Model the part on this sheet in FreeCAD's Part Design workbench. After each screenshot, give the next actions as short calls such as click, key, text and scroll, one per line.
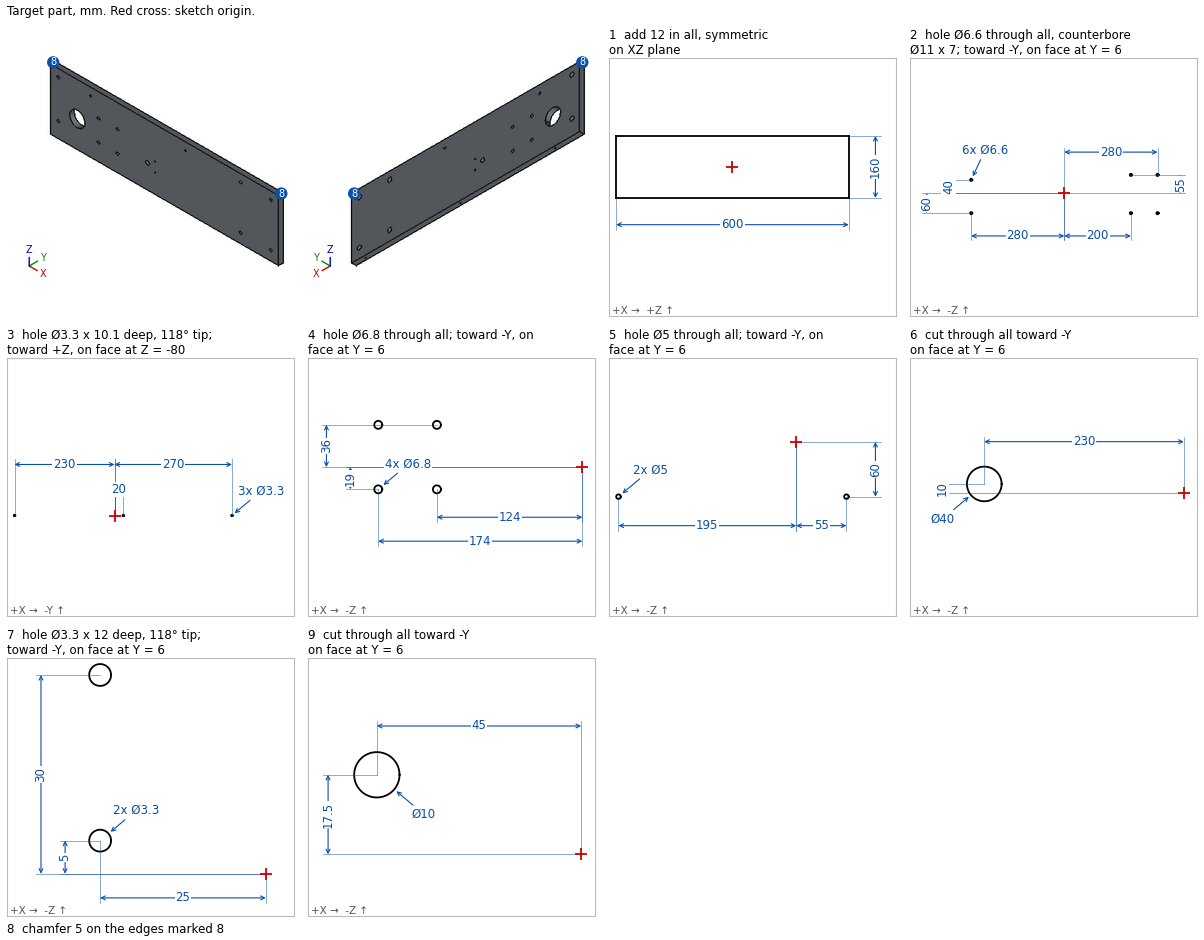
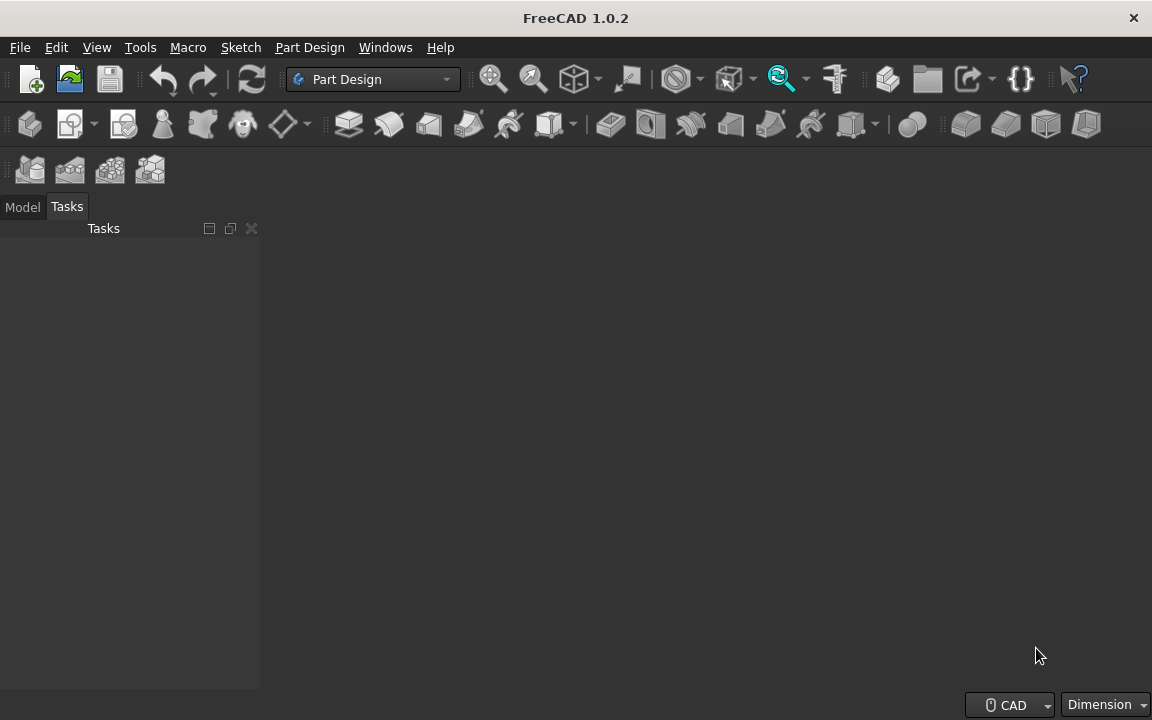
key(ctrl+n)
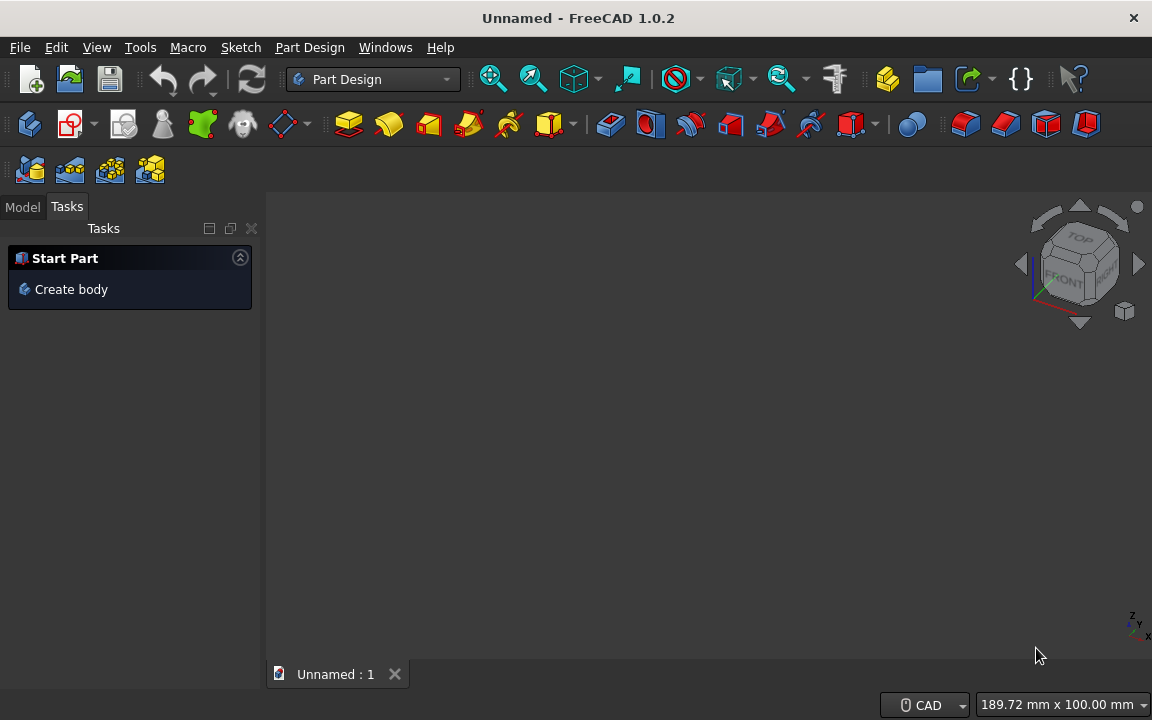
click(70, 124)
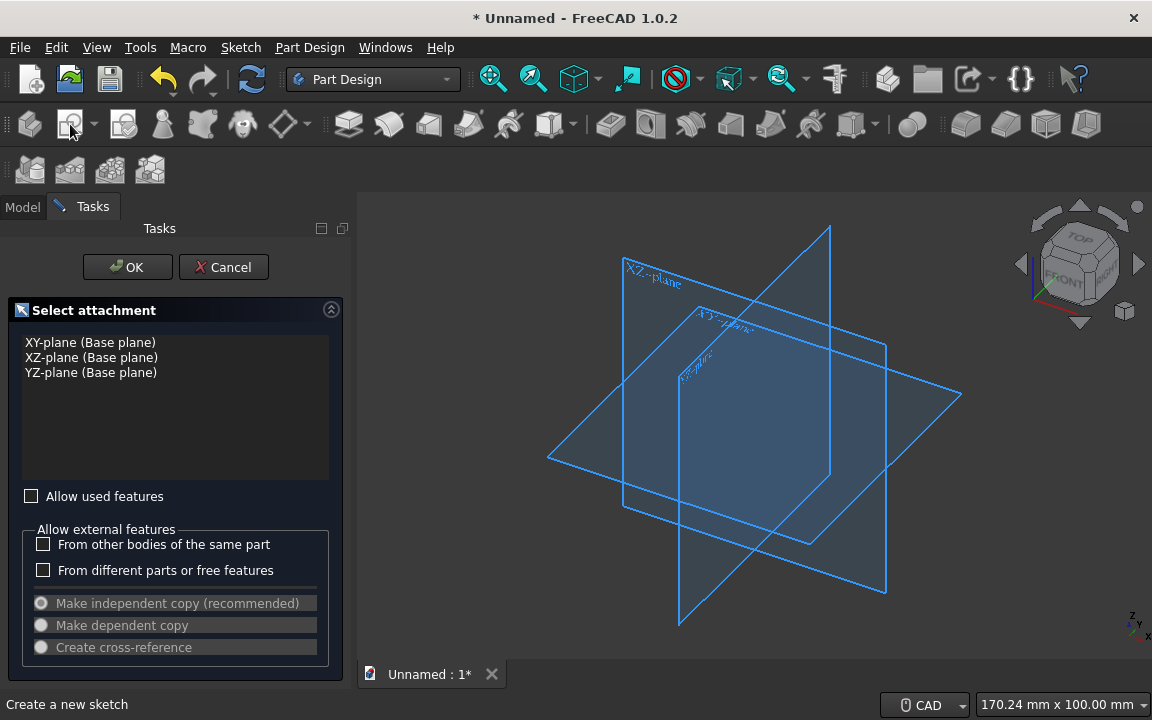
click(82, 358)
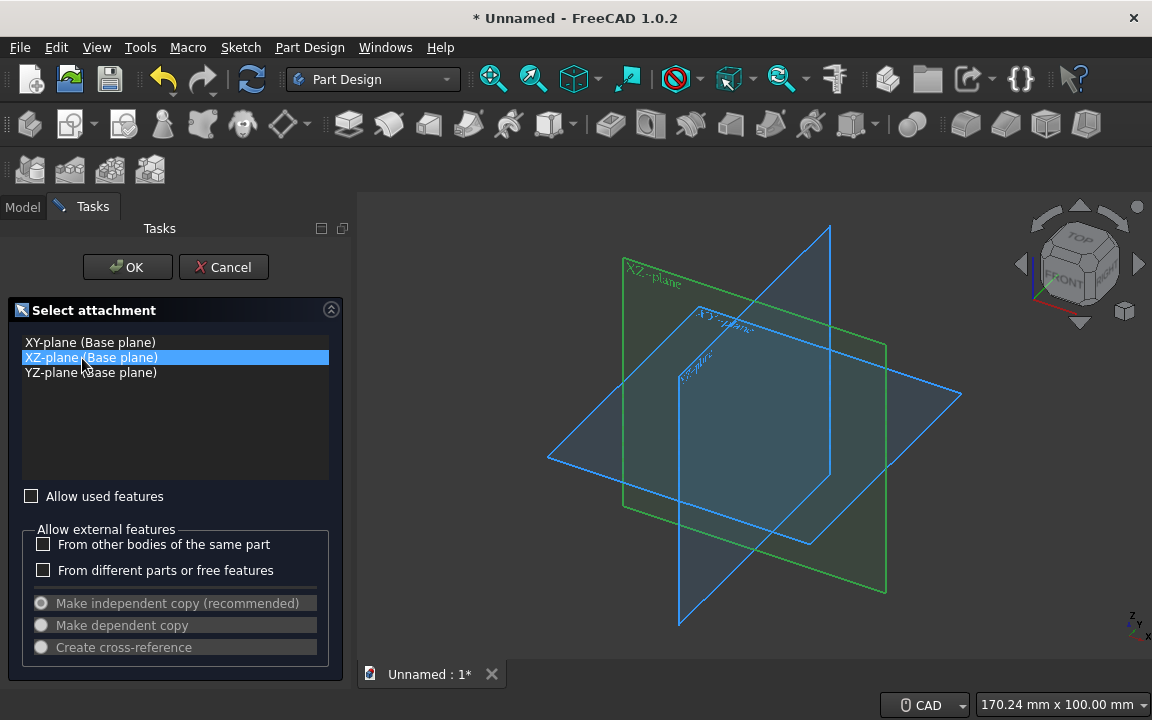
click(128, 267)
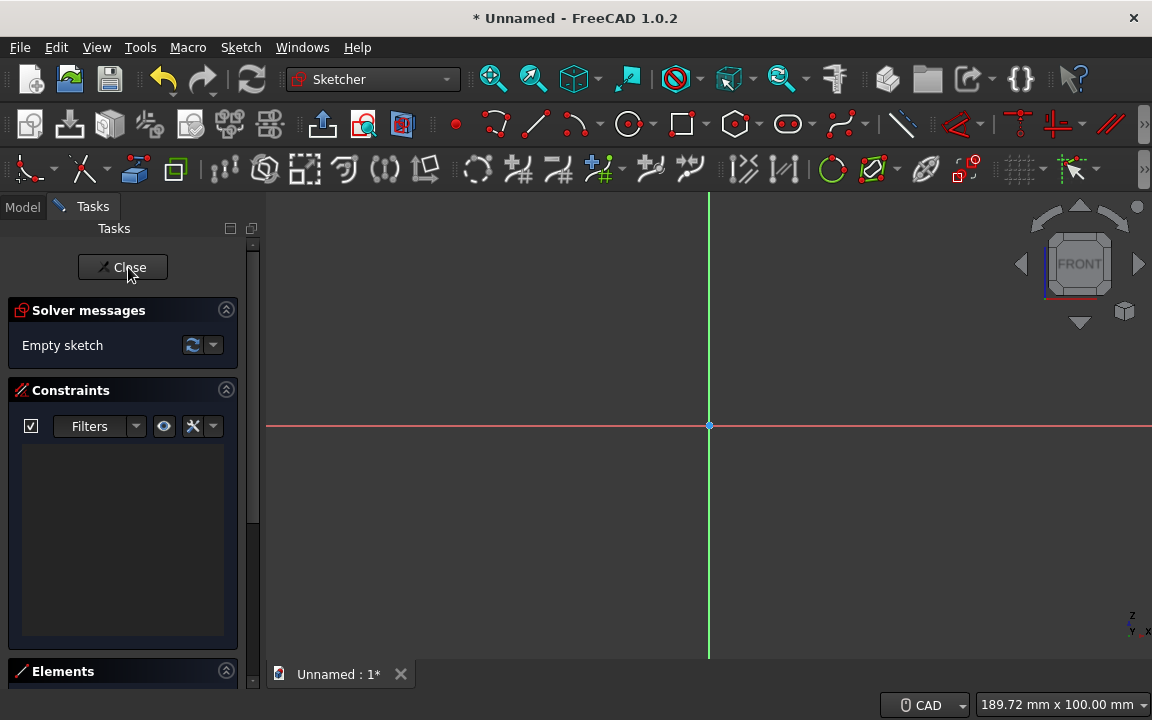
scroll(627, 426, down, 9)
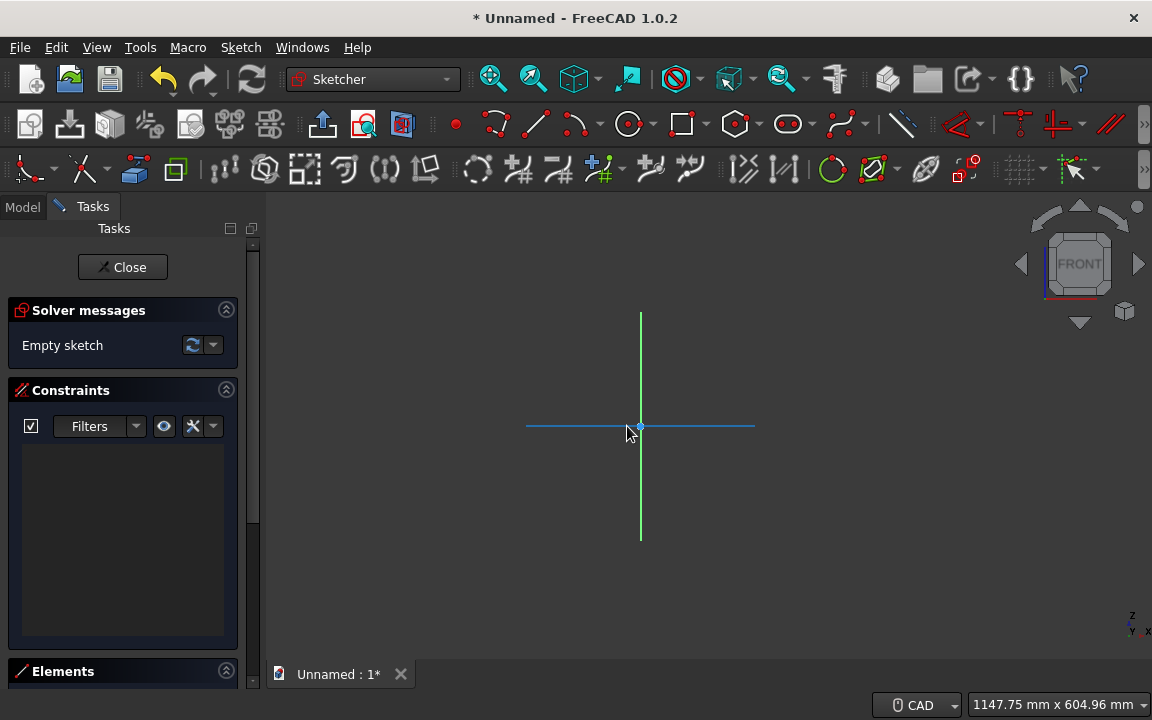
key(g)
key(v)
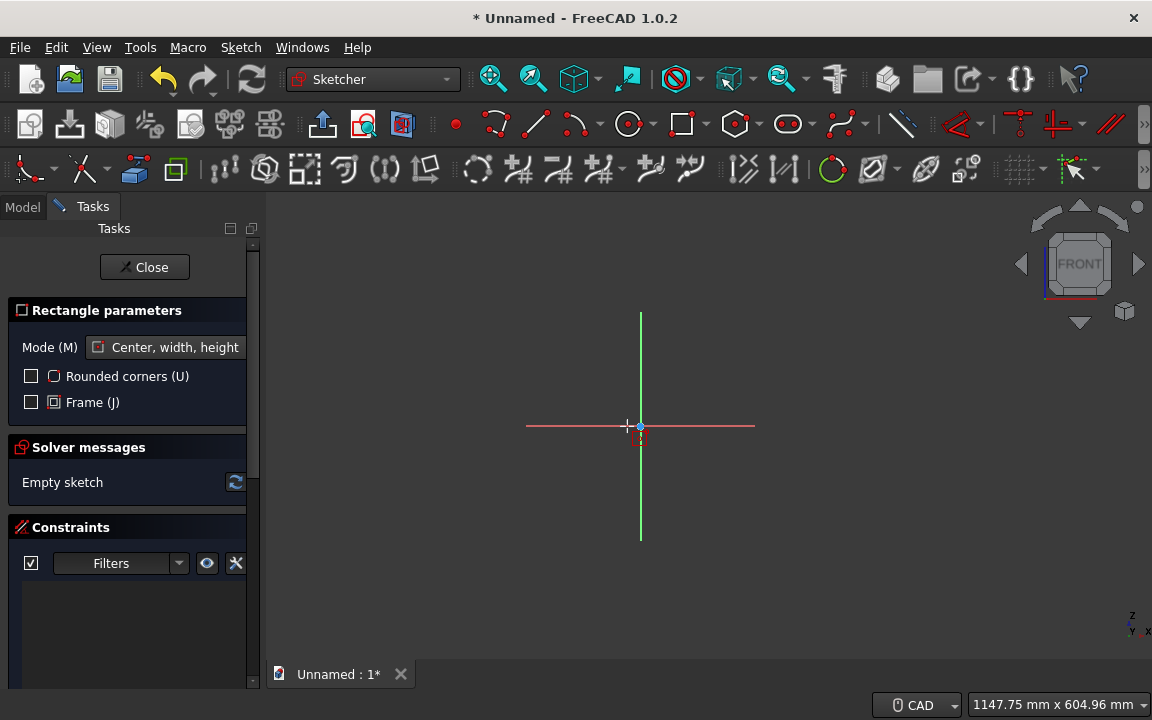
click(641, 426)
move(872, 365)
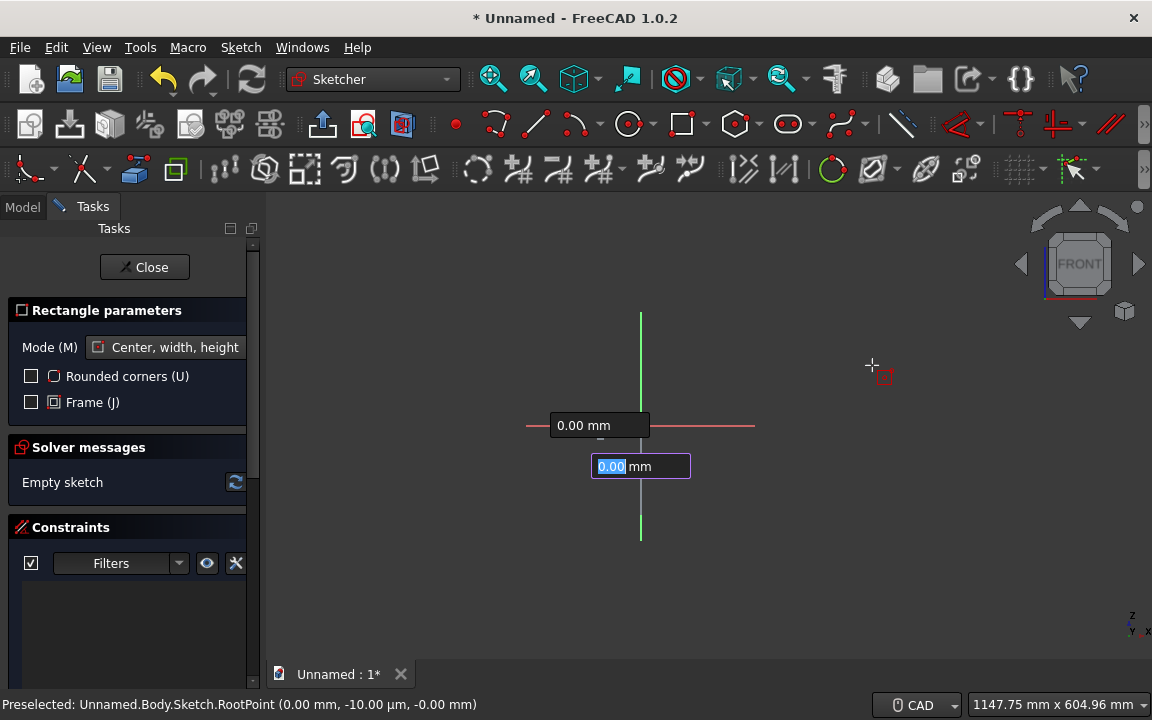
text(600)
key(Tab)
text(160)
key(Return)
key(Escape)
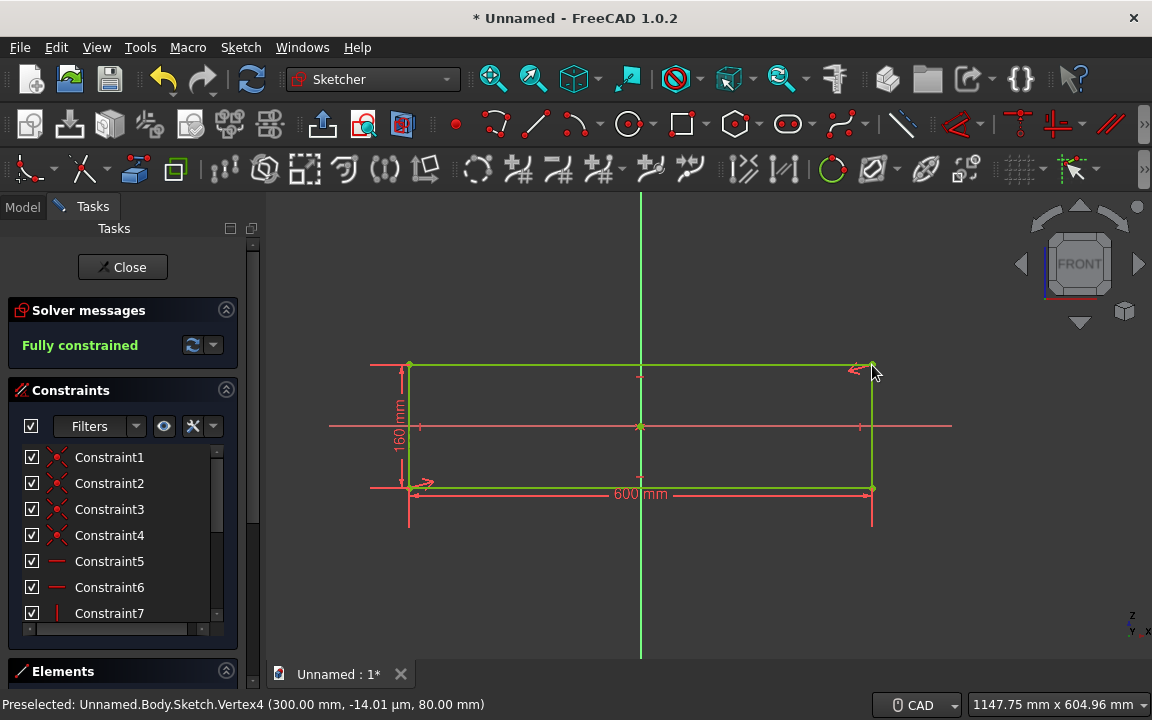
click(123, 267)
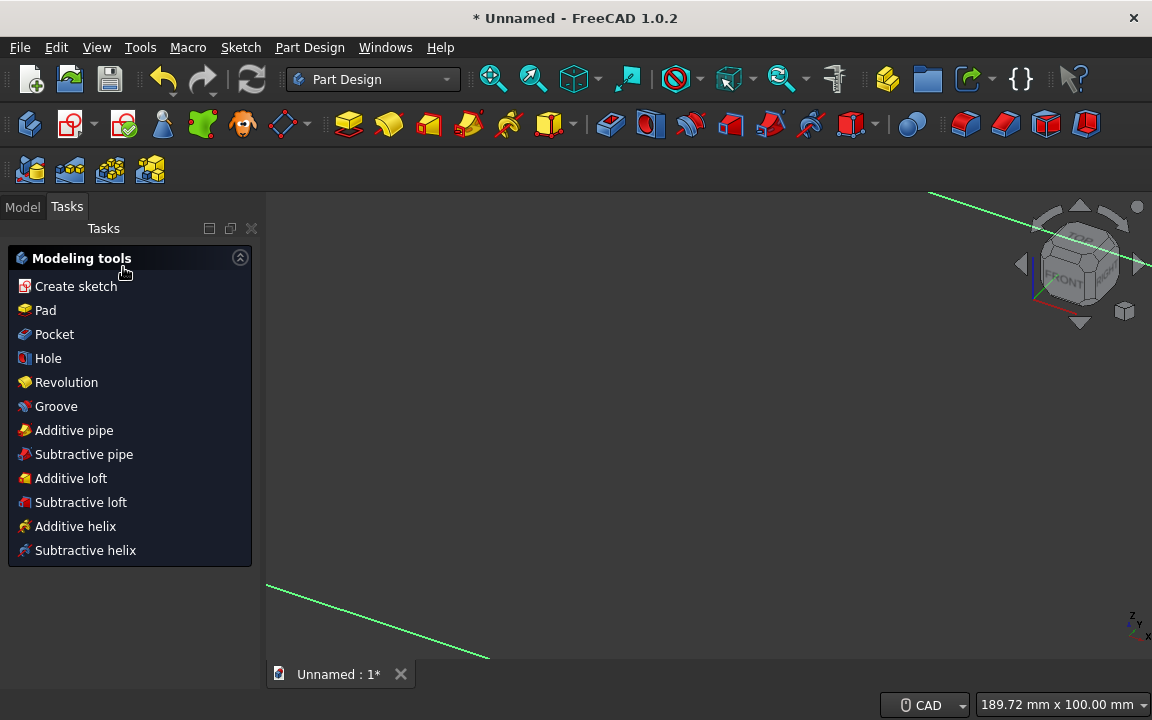
click(350, 124)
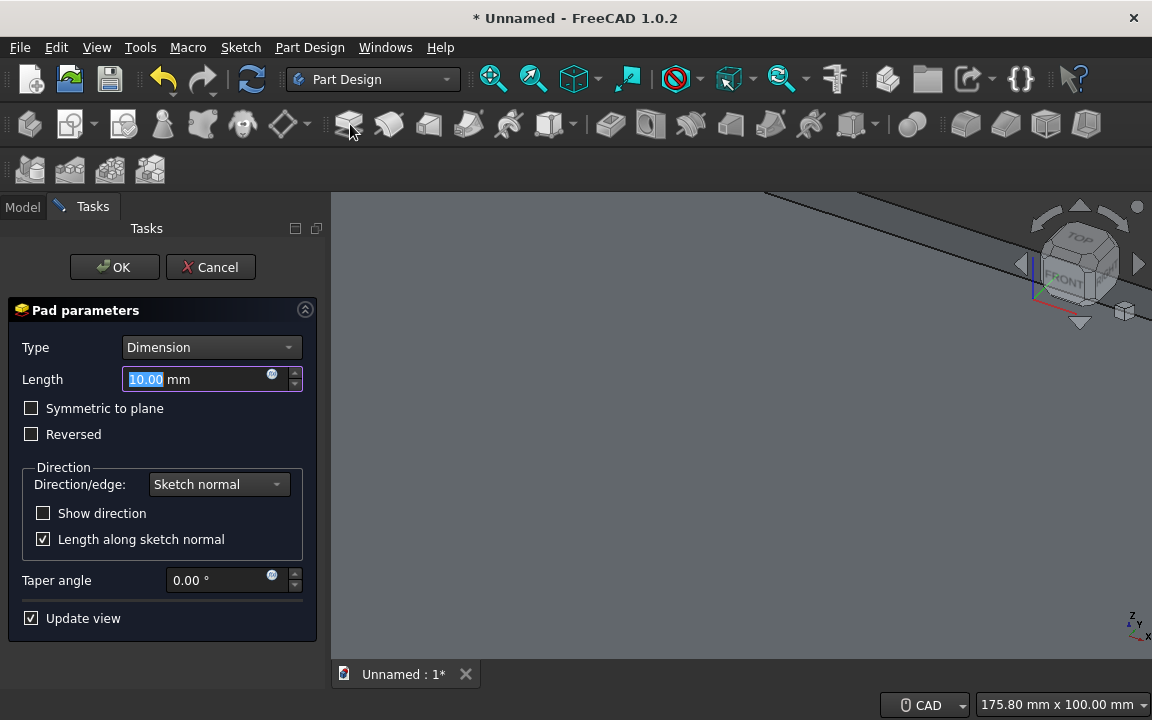
text(12)
key(Tab)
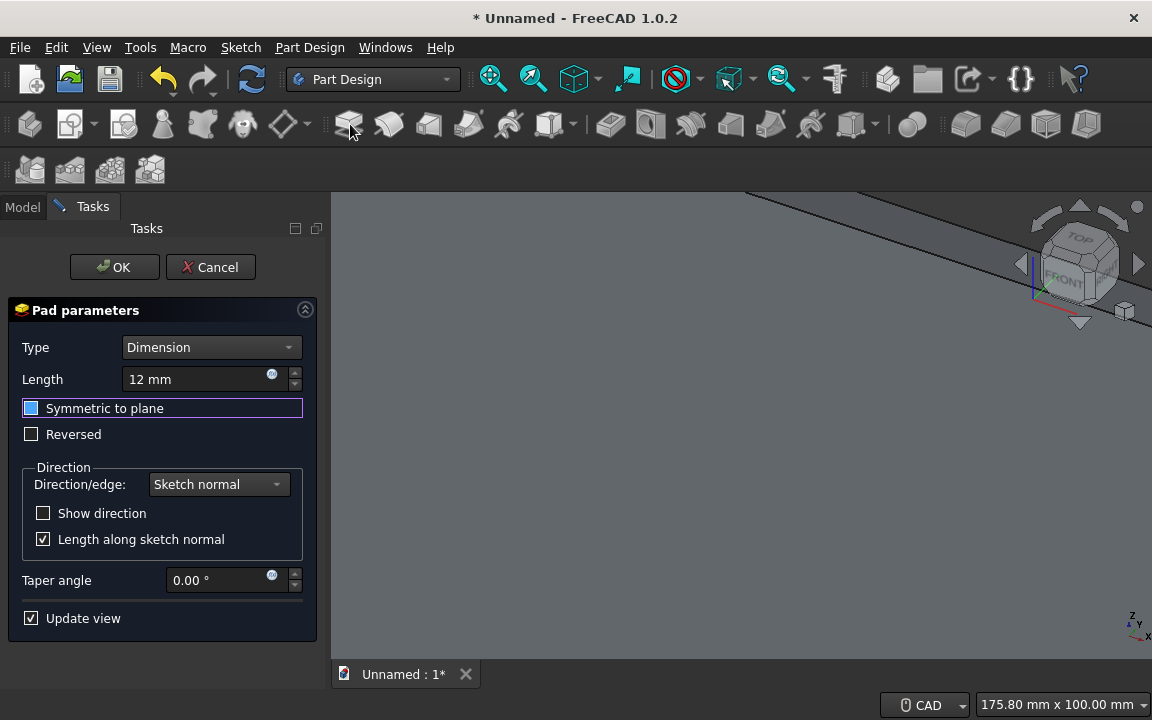
click(30, 408)